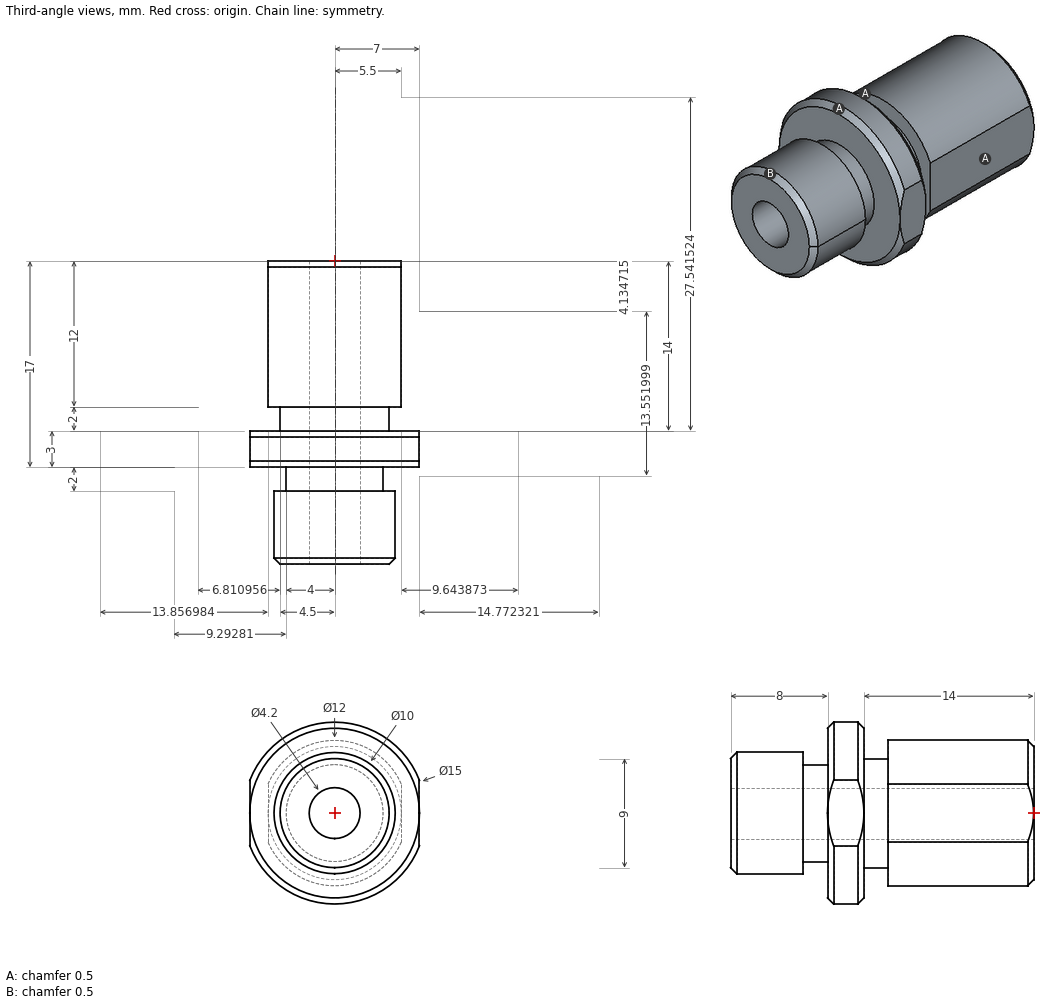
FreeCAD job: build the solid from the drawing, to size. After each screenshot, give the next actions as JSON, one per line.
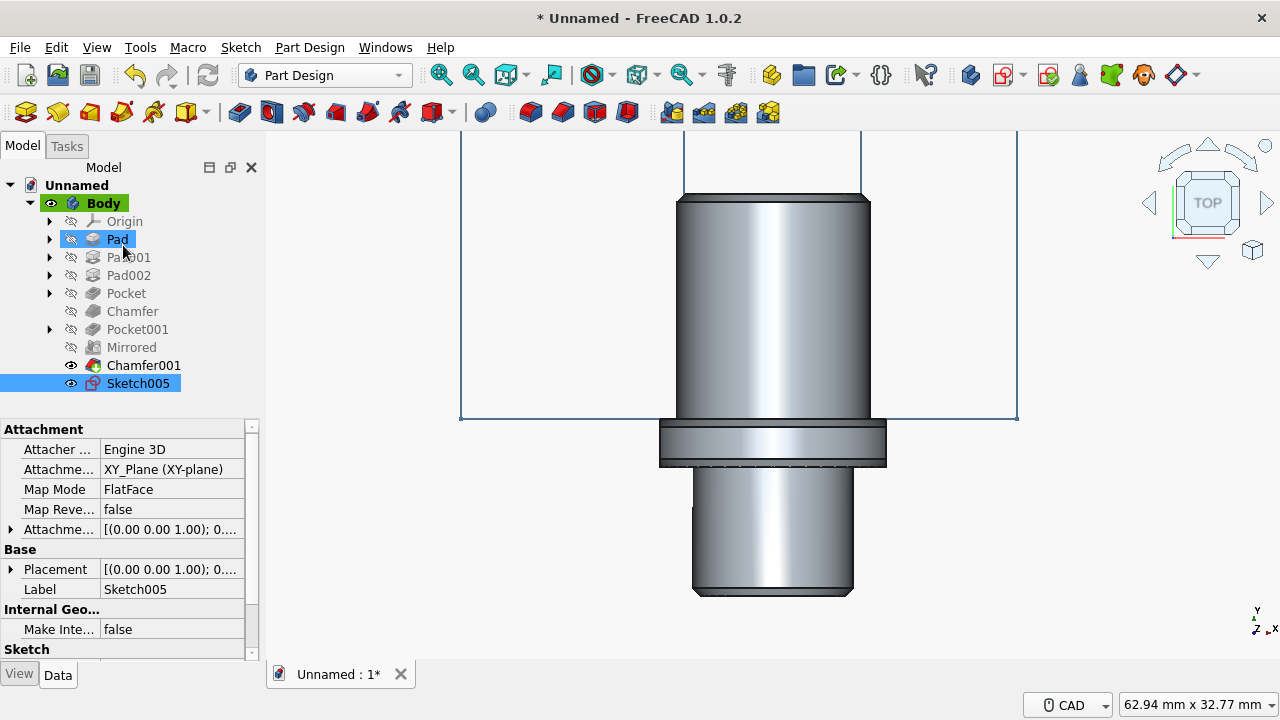
{"action": "left_click", "coordinate": [240, 112]}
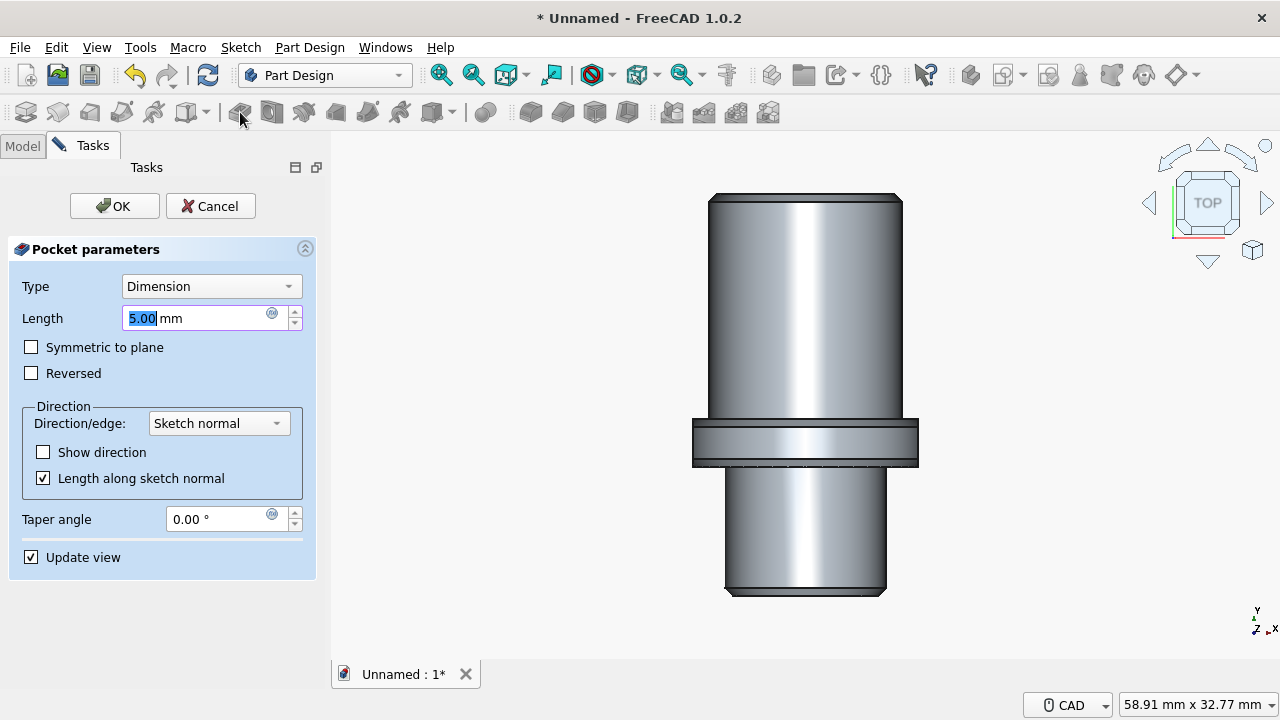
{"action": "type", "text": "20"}
{"action": "key", "text": "Tab"}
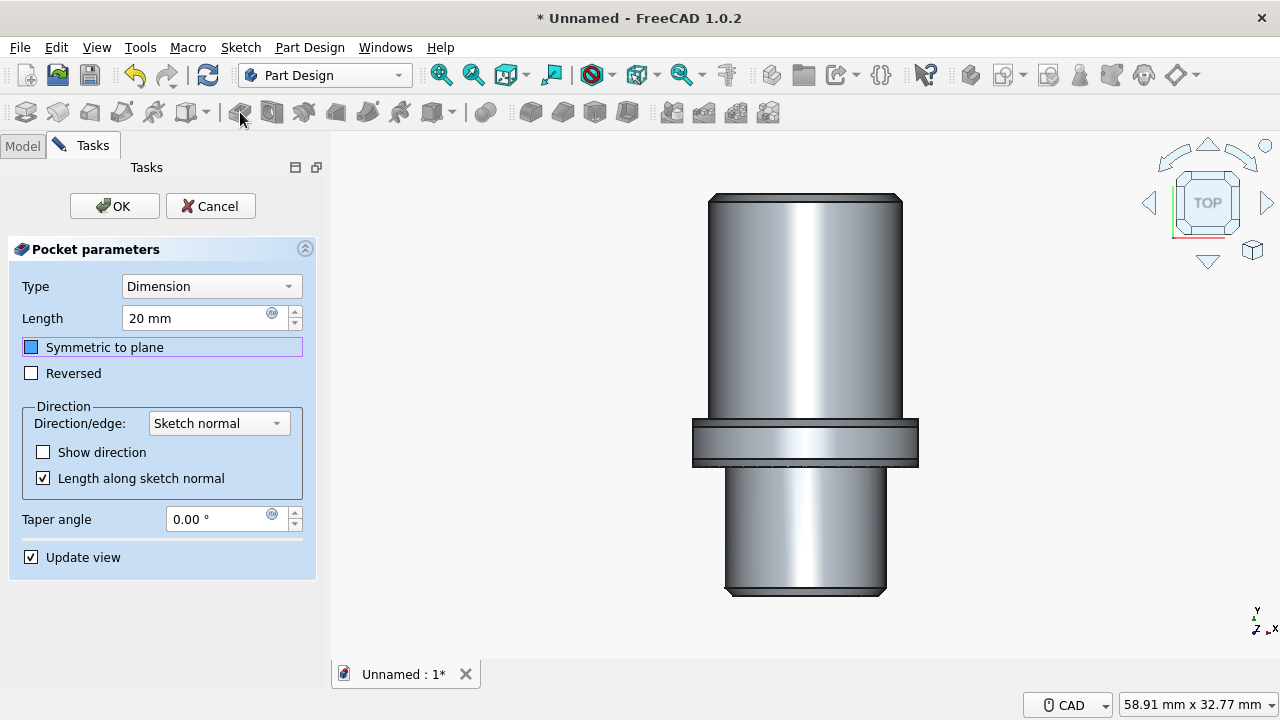
{"action": "left_click", "coordinate": [30, 347]}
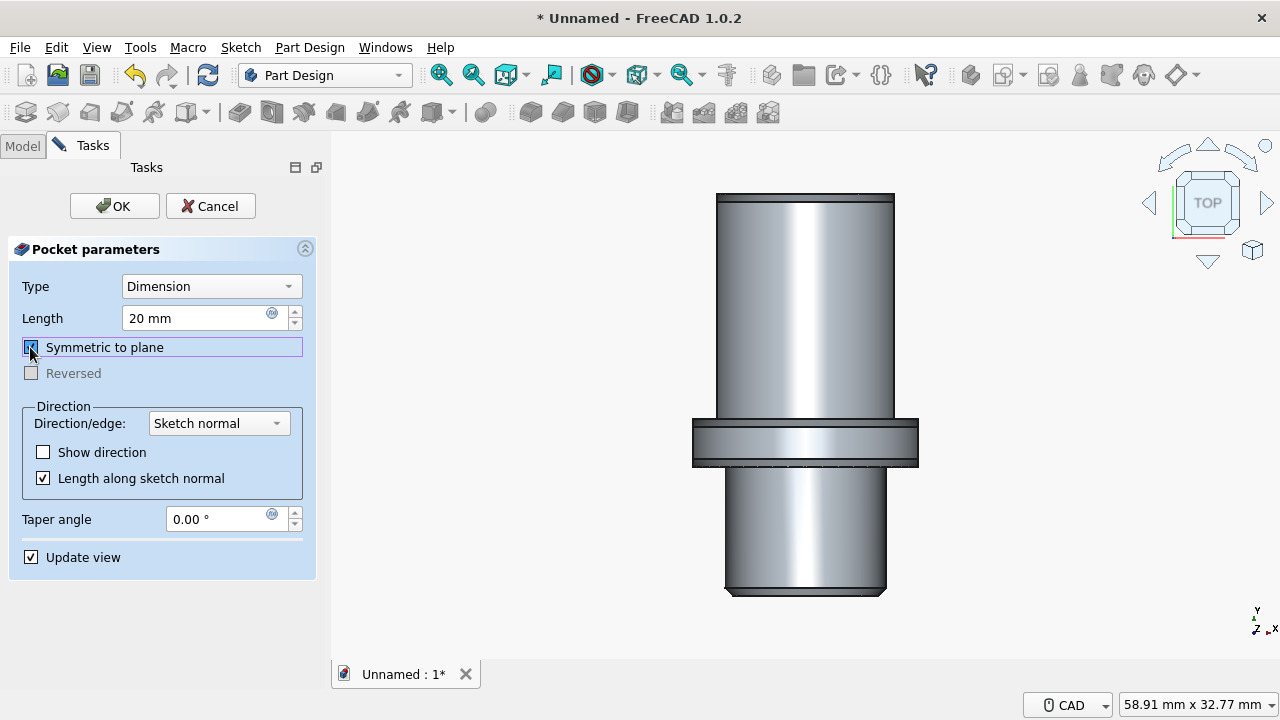
{"action": "left_click", "coordinate": [115, 206]}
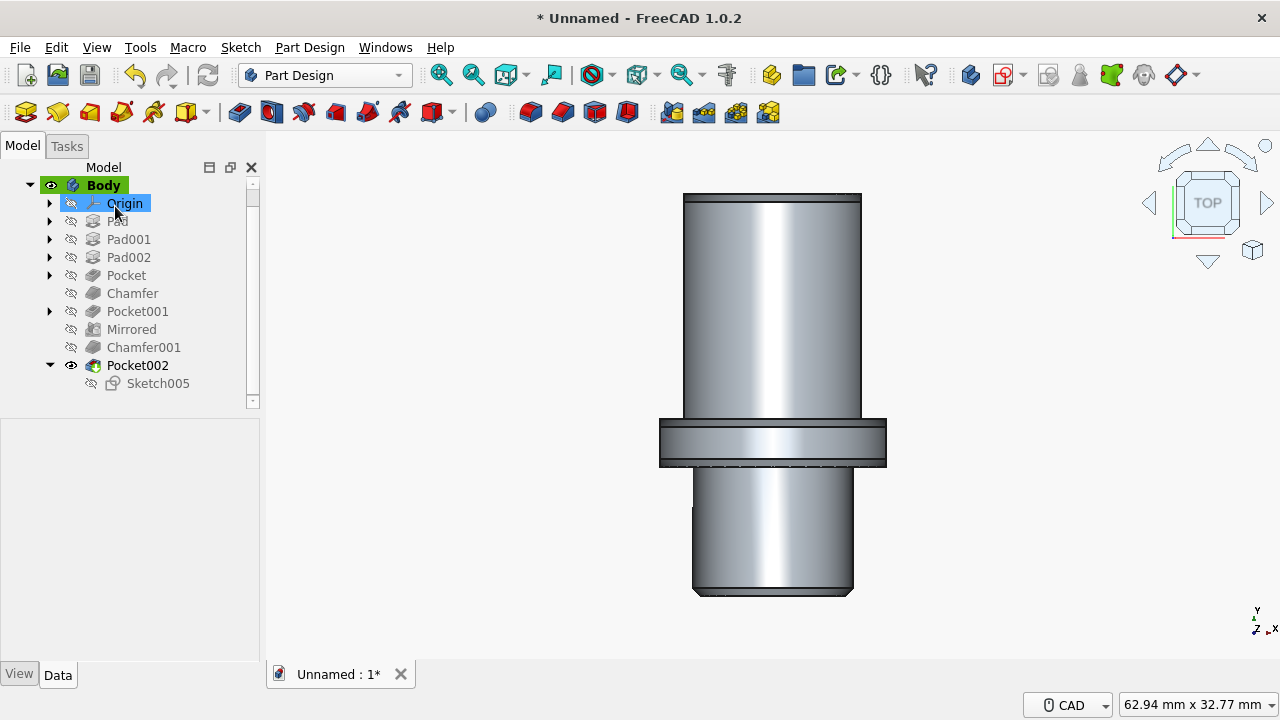
{"action": "left_click", "coordinate": [1004, 76]}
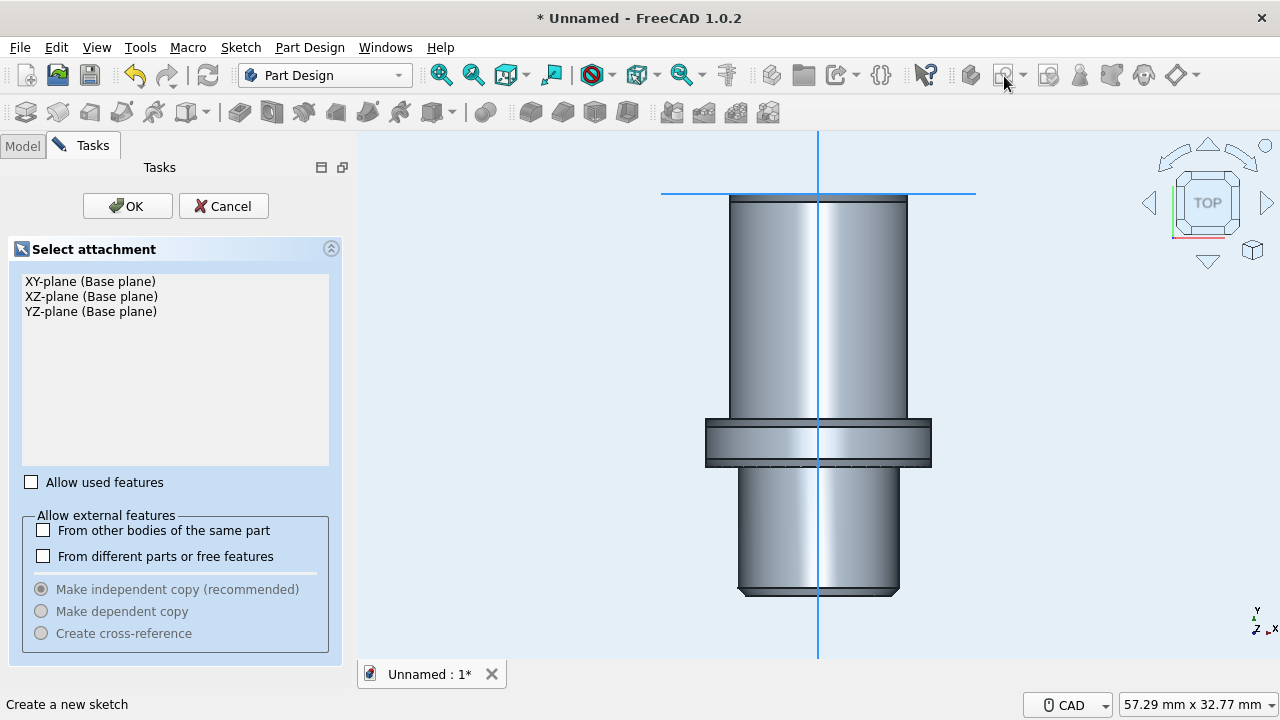
{"action": "left_click", "coordinate": [82, 282]}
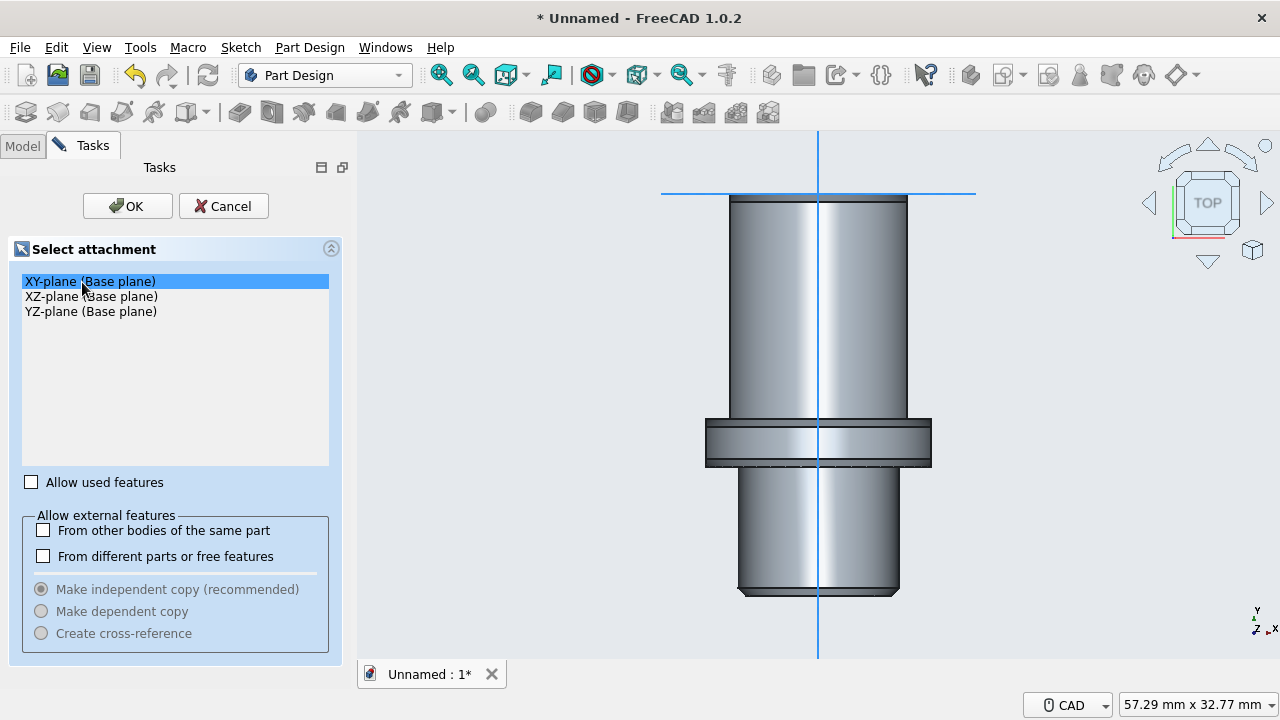
{"action": "left_click", "coordinate": [128, 206]}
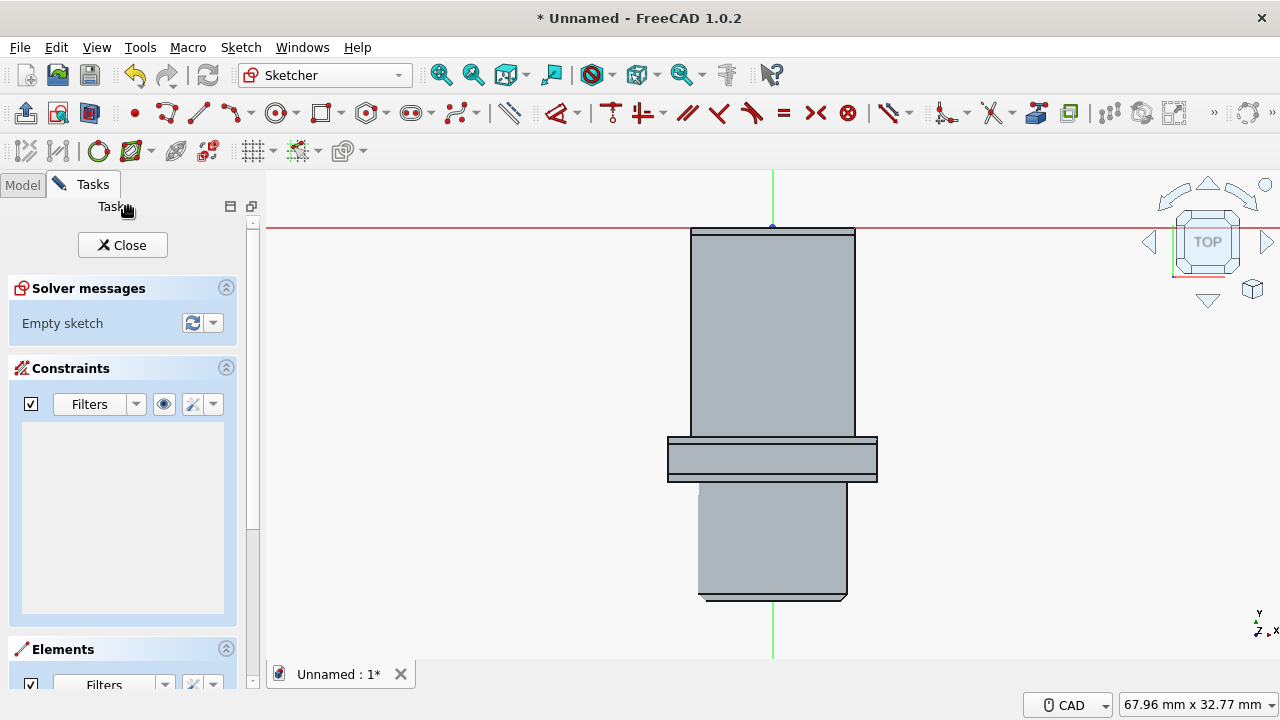
{"action": "key", "text": "q s"}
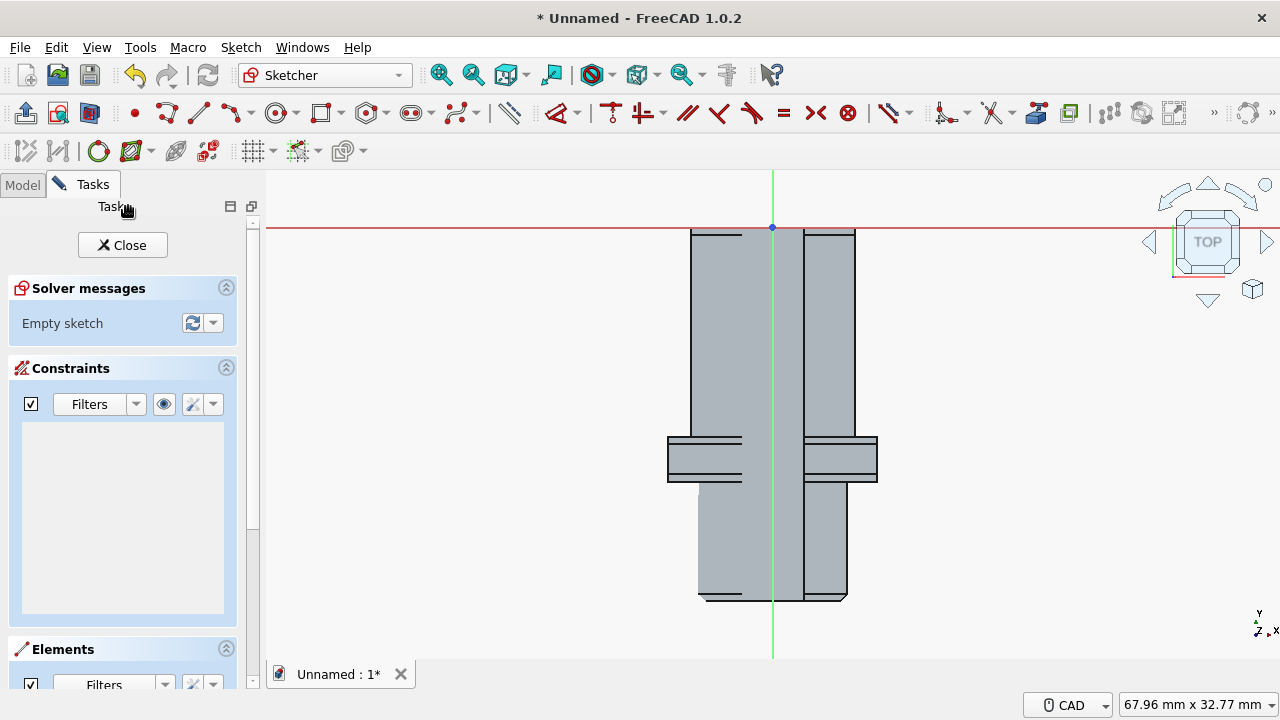
{"action": "key", "text": "g r"}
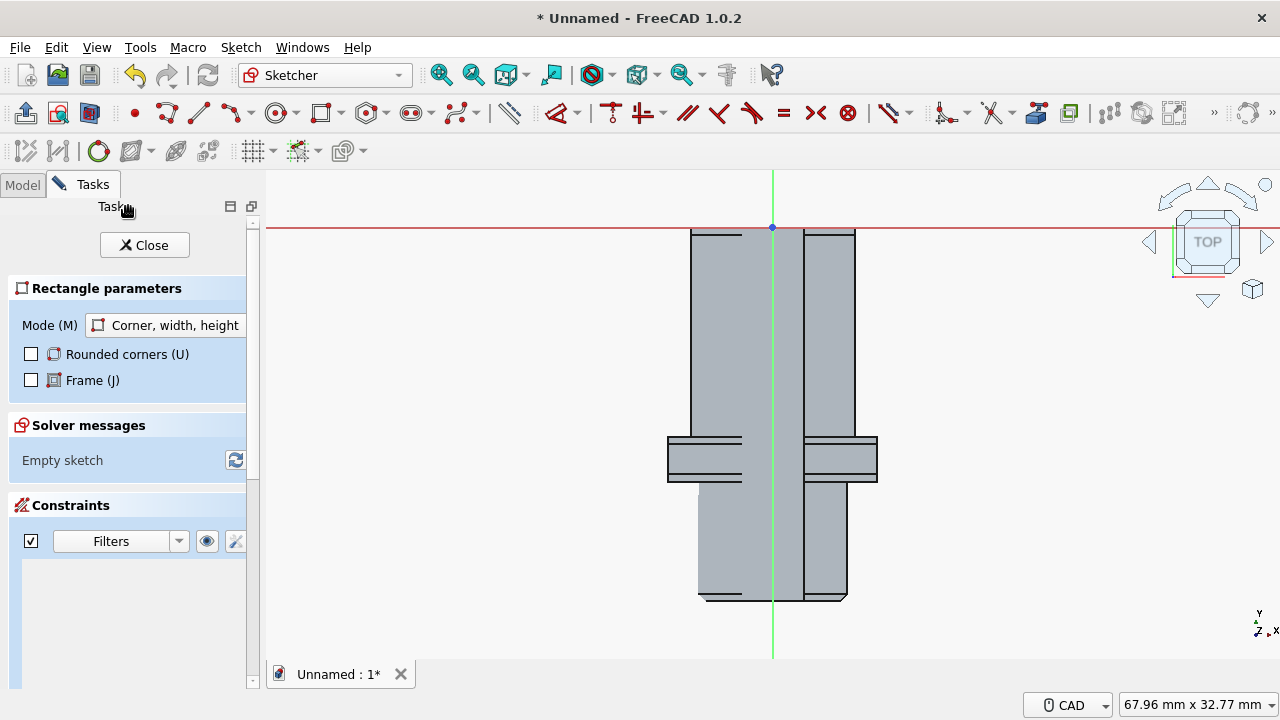
{"action": "left_click", "coordinate": [575, 482]}
{"action": "left_click", "coordinate": [713, 511]}
{"action": "key", "text": "Escape"}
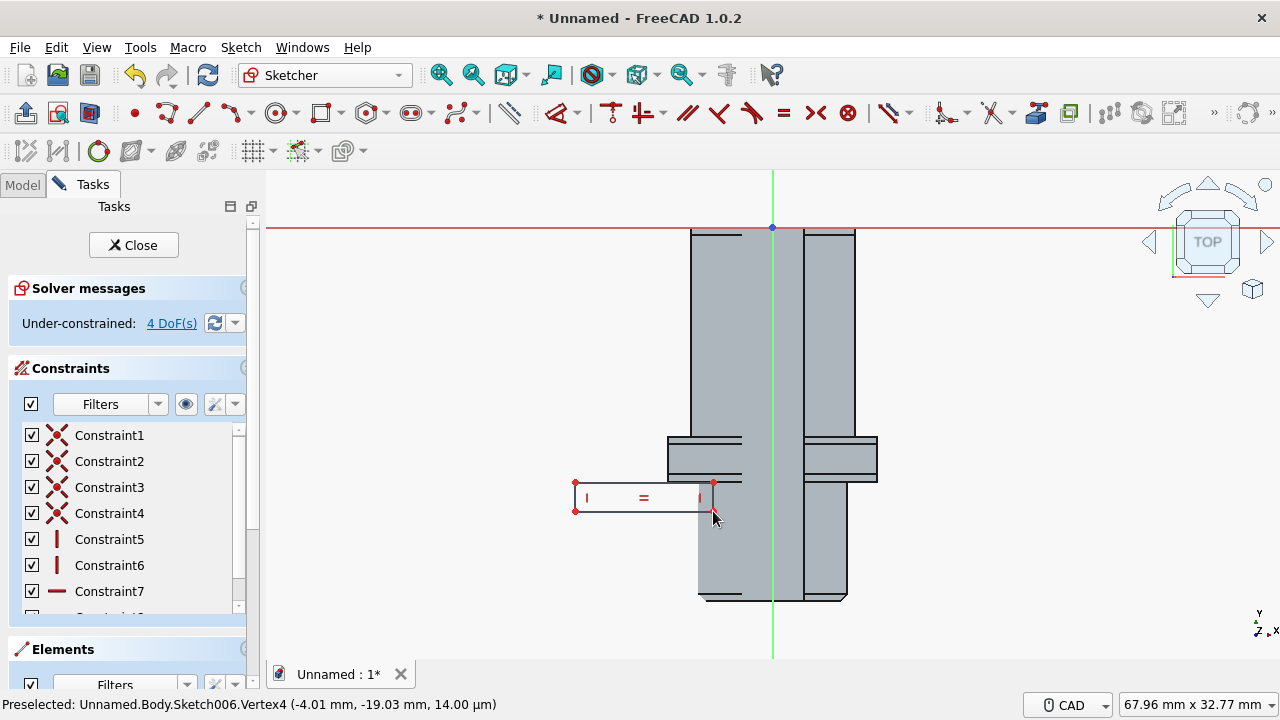
{"action": "key", "text": "d"}